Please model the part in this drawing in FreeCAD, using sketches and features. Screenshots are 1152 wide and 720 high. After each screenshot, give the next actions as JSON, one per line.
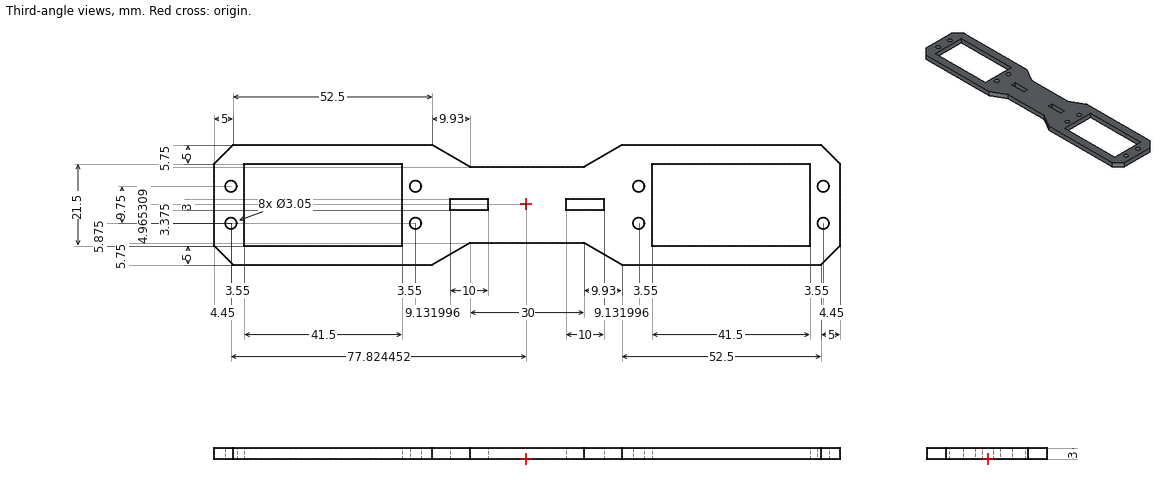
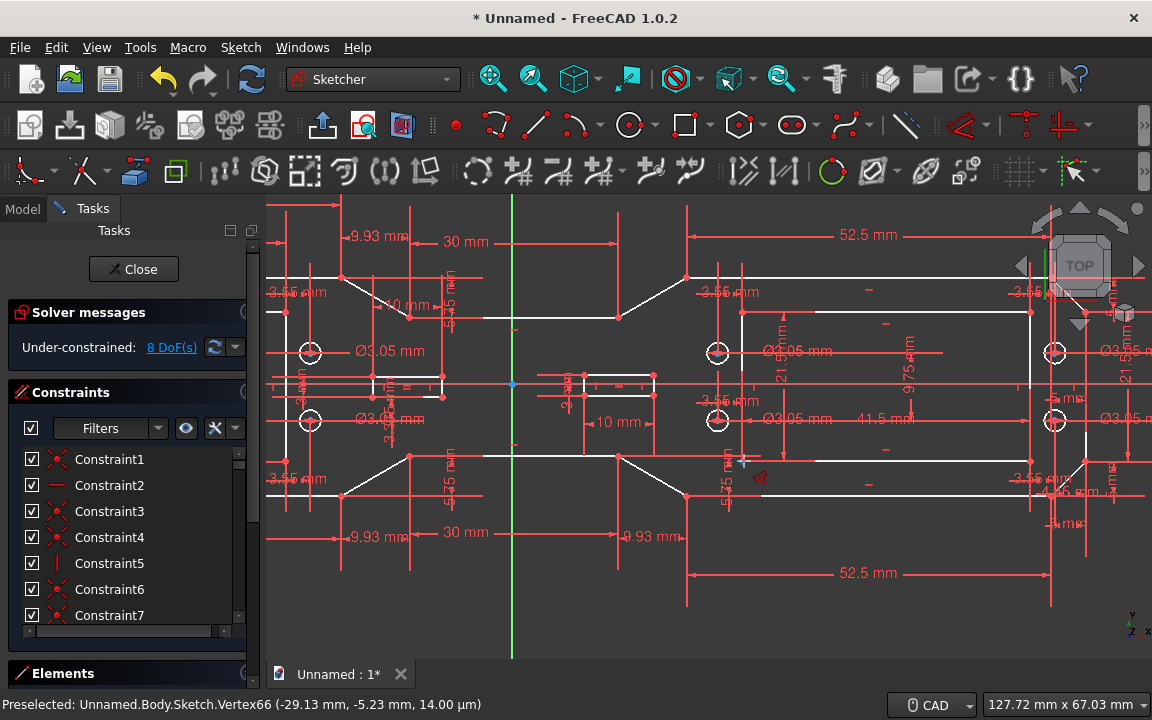
{"action": "left_click", "coordinate": [742, 461]}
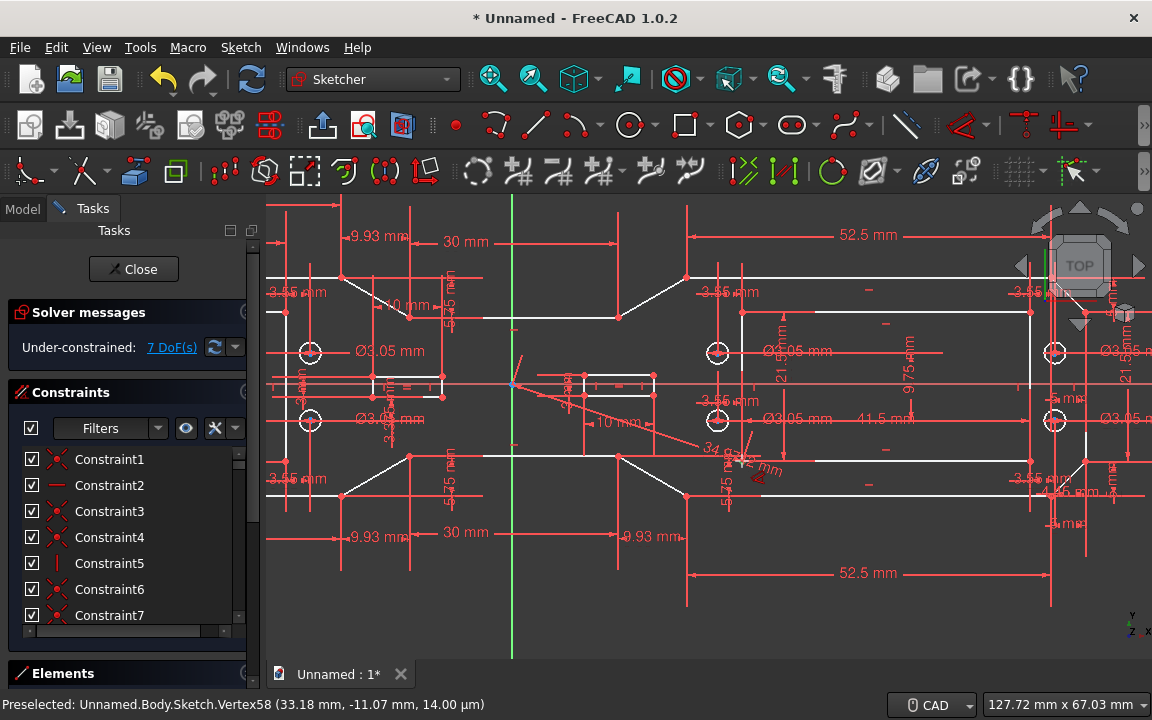
{"action": "left_click", "coordinate": [718, 421]}
{"action": "left_click", "coordinate": [776, 441]}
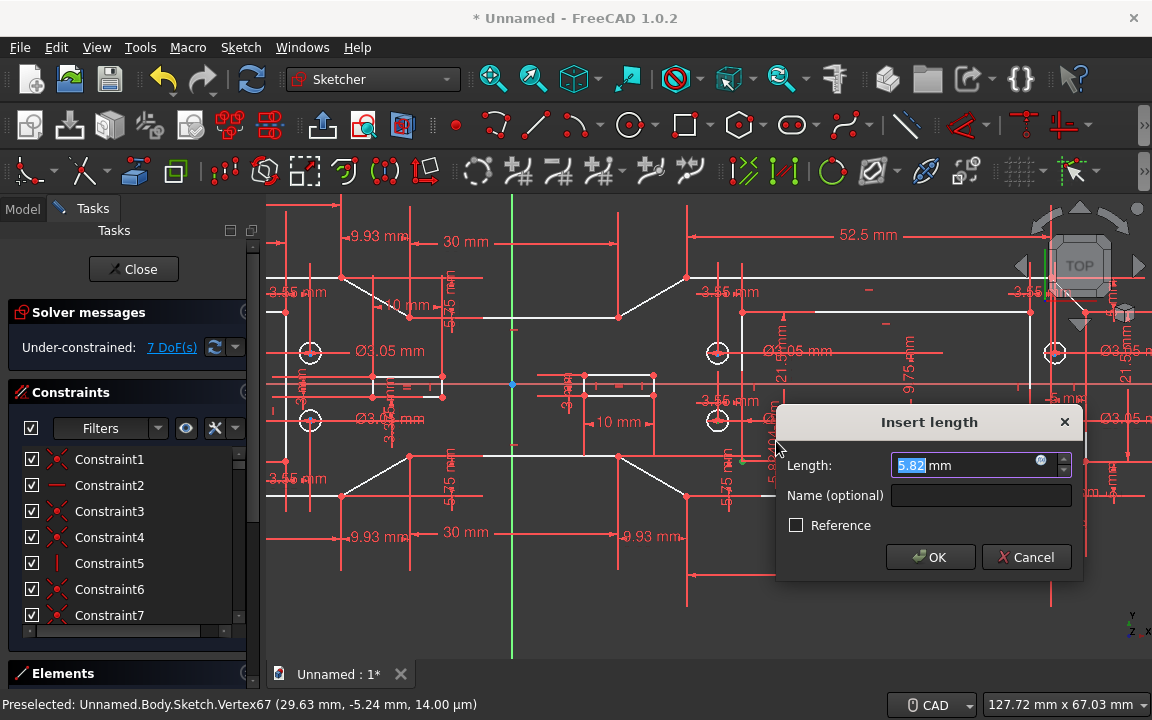
{"action": "type", "text": "5.875"}
{"action": "key", "text": "Return"}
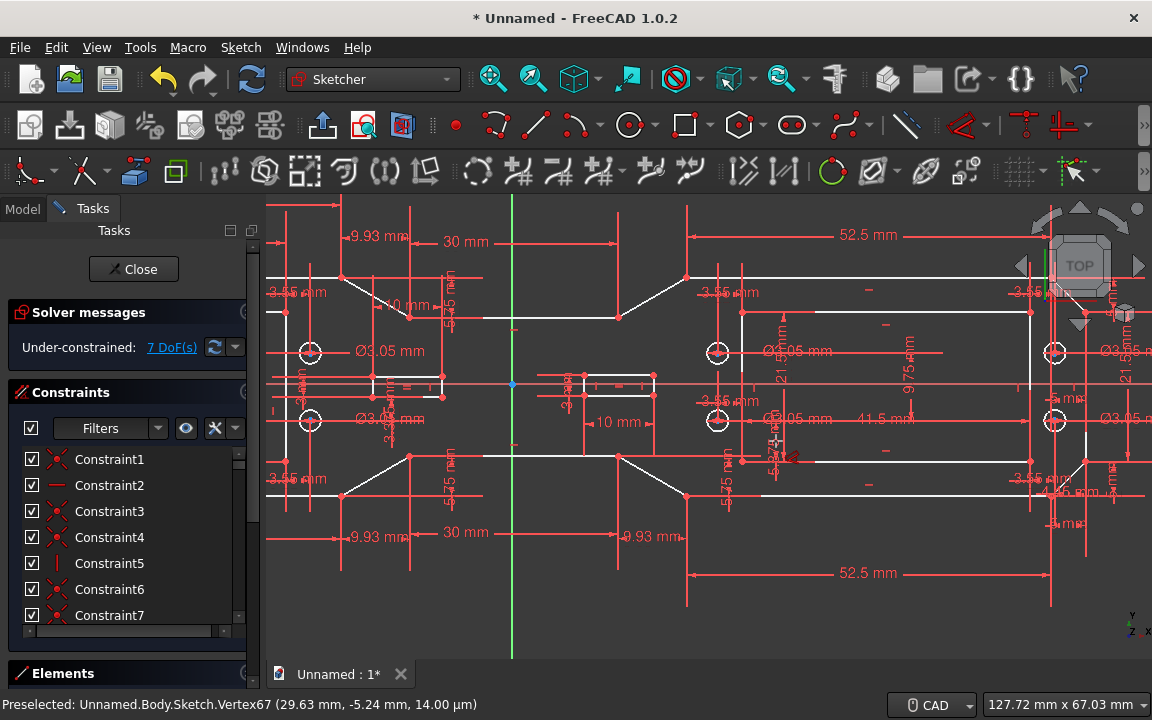
{"action": "scroll", "coordinate": [654, 396], "scroll_direction": "up", "scroll_amount": 3}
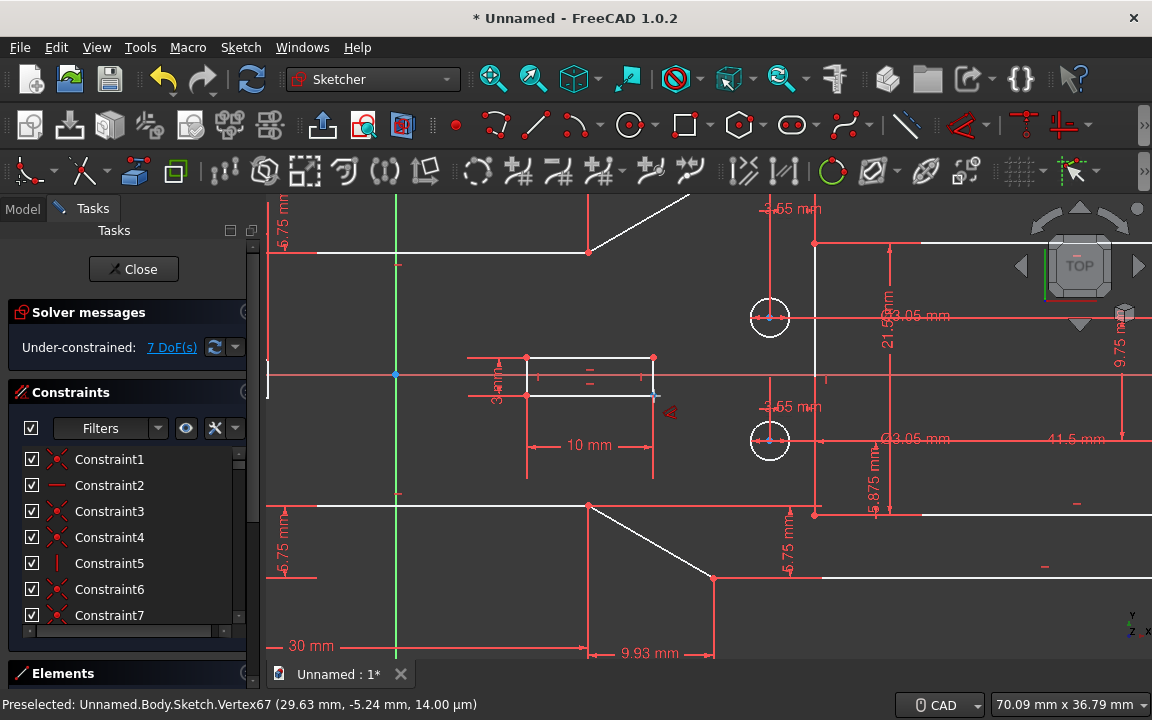
{"action": "left_click", "coordinate": [653, 396]}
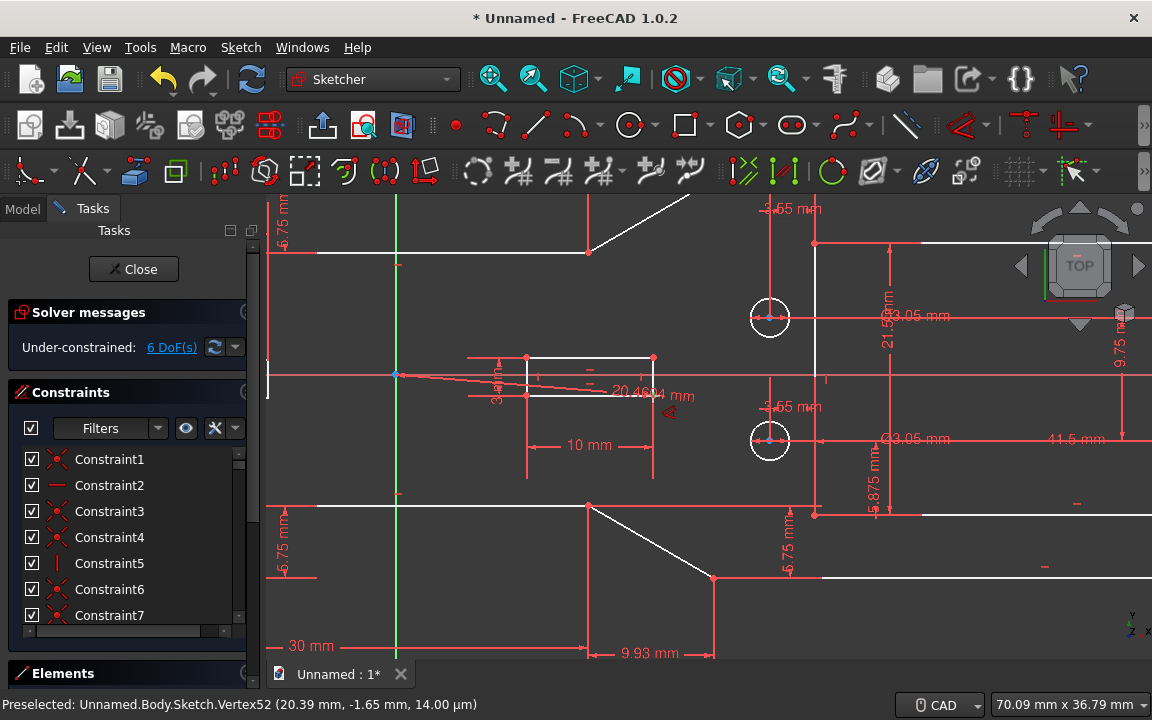
{"action": "left_click", "coordinate": [770, 441]}
{"action": "left_click", "coordinate": [619, 418]}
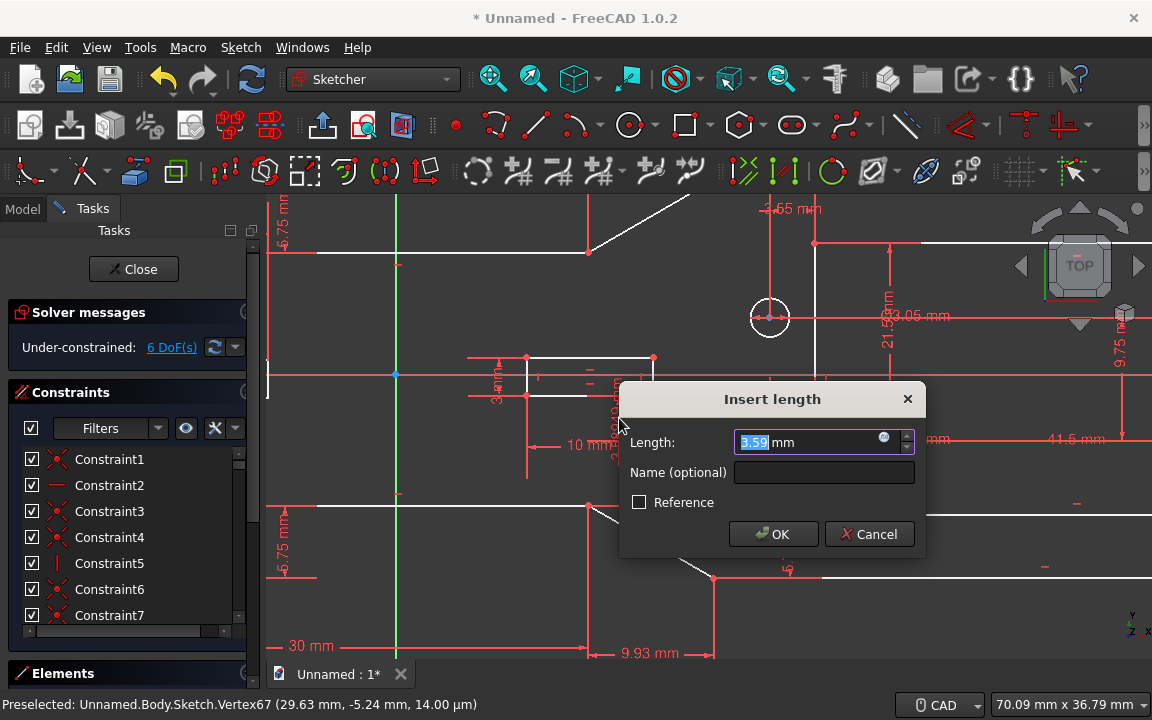
{"action": "type", "text": "3.375"}
{"action": "key", "text": "Return"}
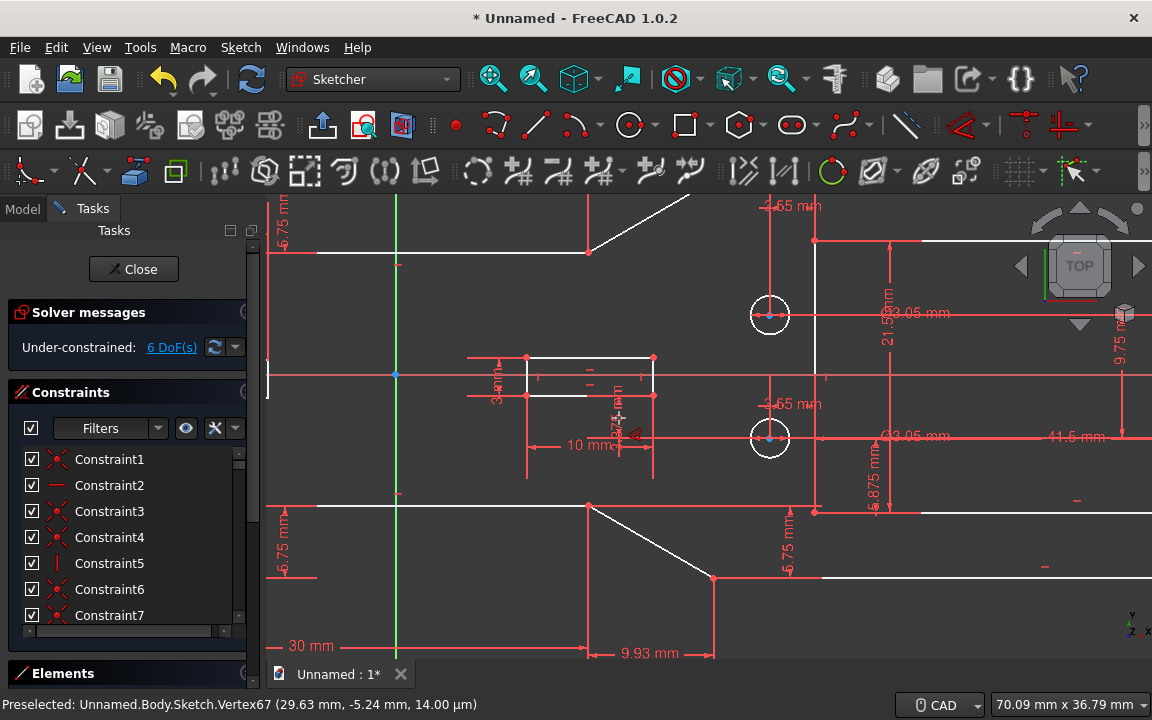
{"action": "scroll", "coordinate": [720, 443], "scroll_direction": "down", "scroll_amount": 7}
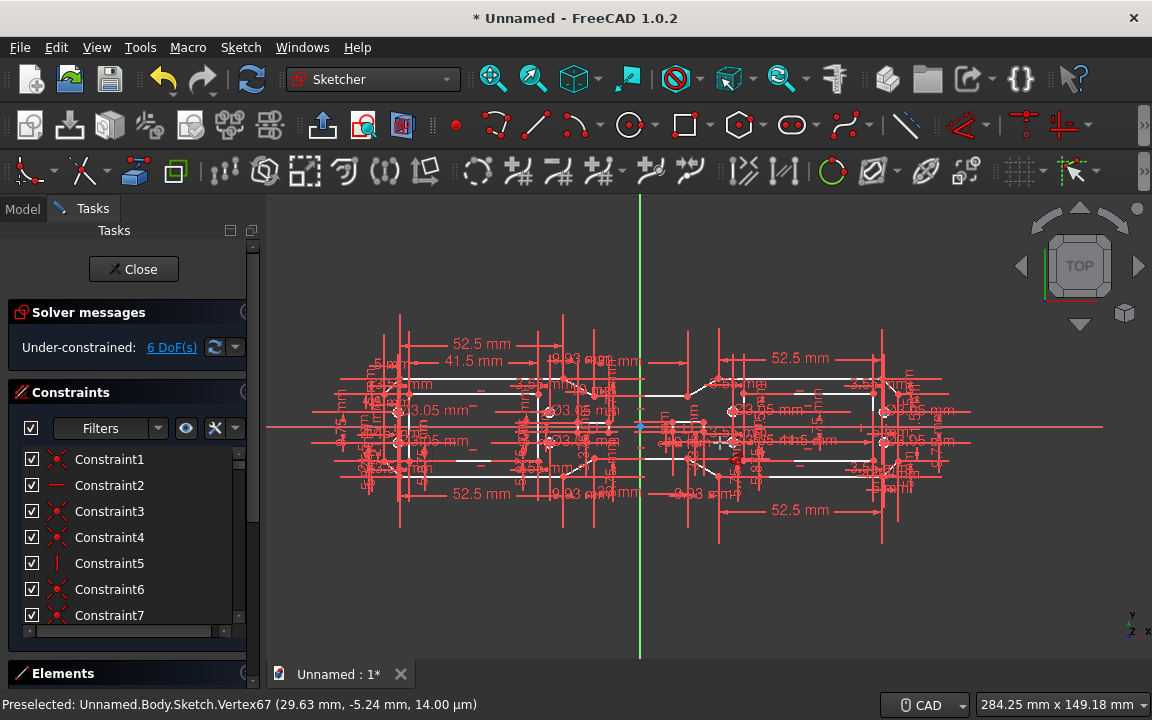
{"action": "scroll", "coordinate": [873, 461], "scroll_direction": "up", "scroll_amount": 4}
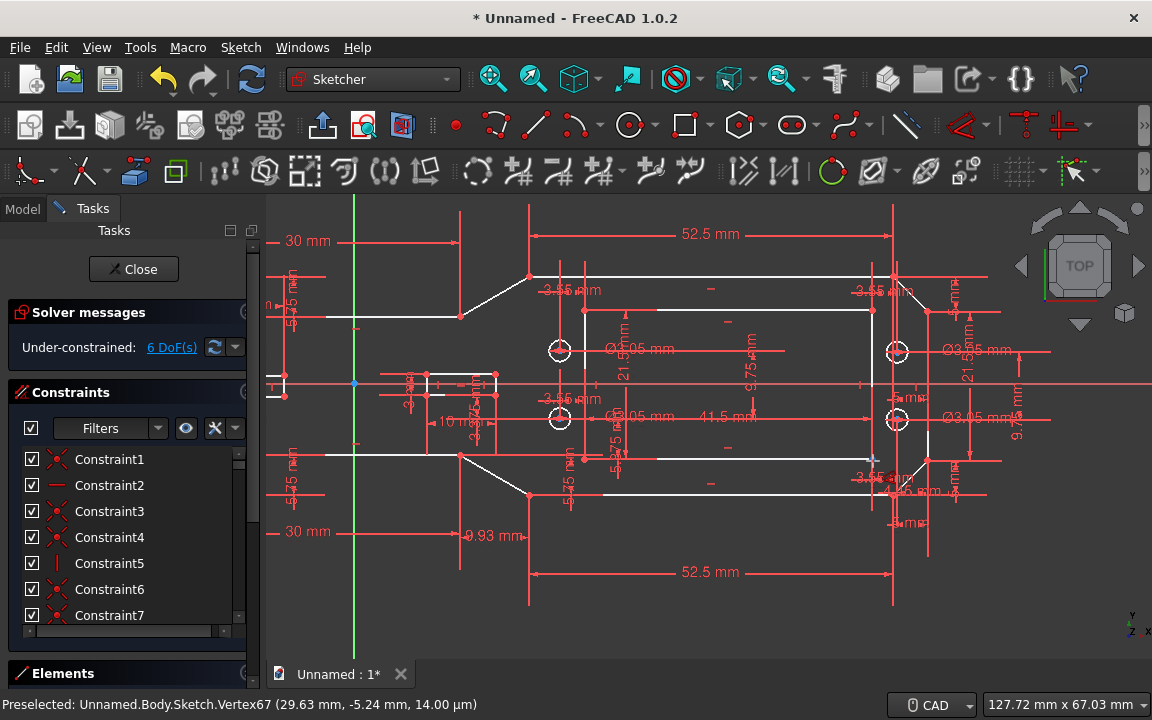
{"action": "left_click", "coordinate": [872, 459]}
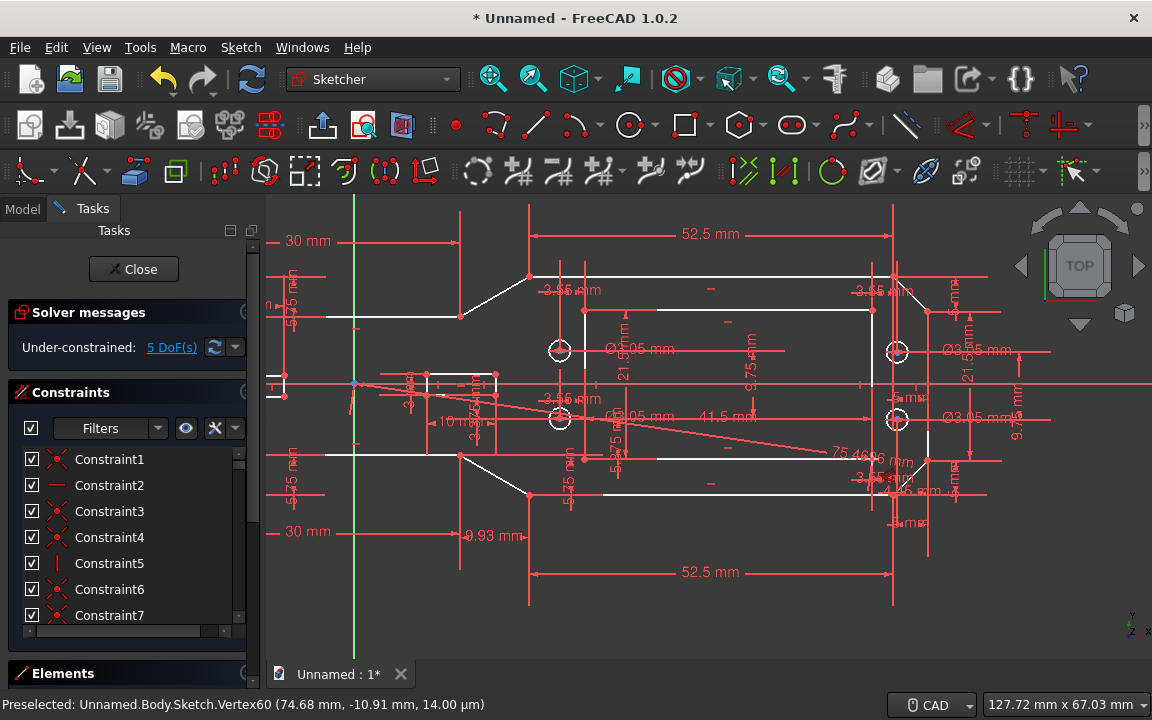
{"action": "left_click", "coordinate": [897, 420]}
{"action": "left_click", "coordinate": [838, 440]}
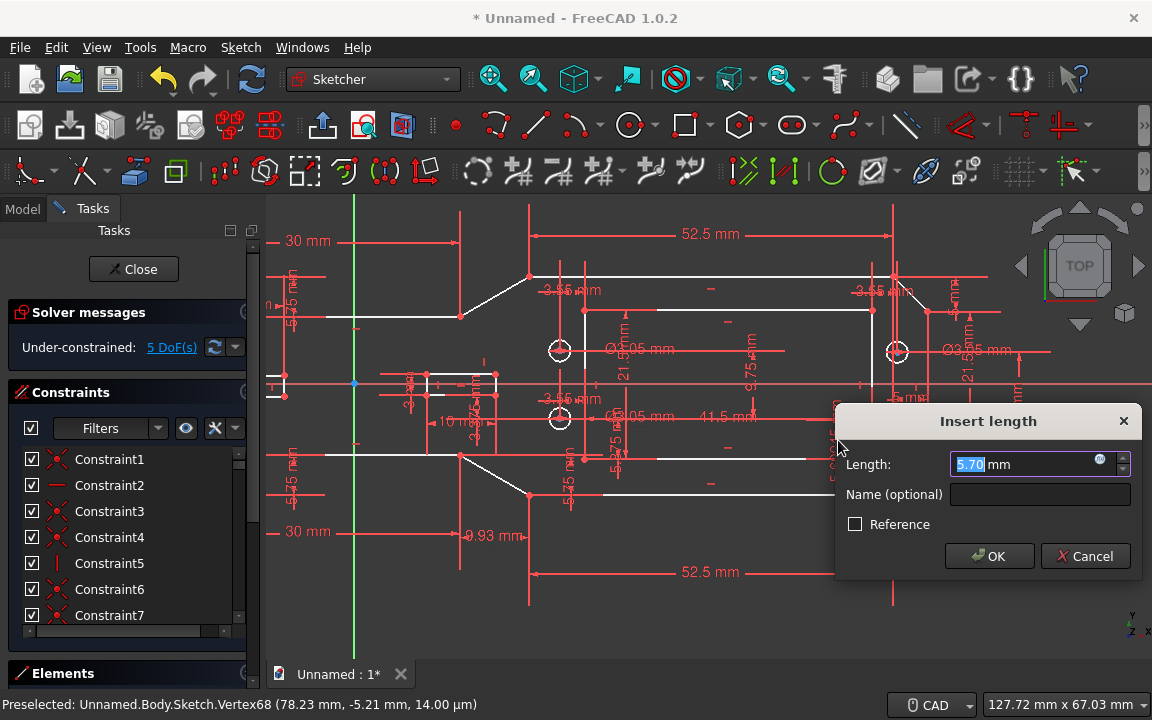
{"action": "type", "text": "5.875"}
{"action": "key", "text": "Return"}